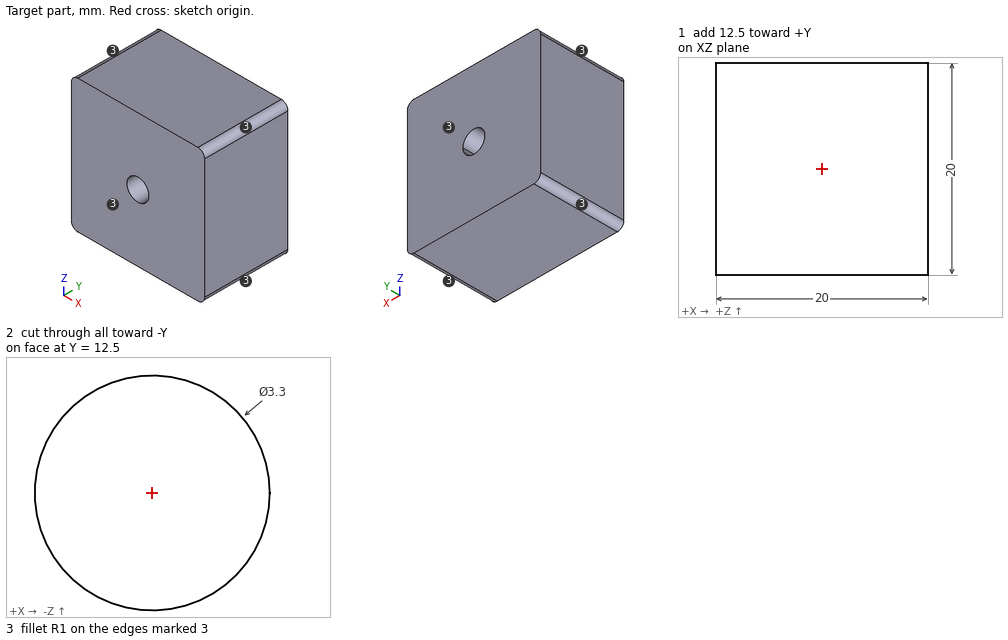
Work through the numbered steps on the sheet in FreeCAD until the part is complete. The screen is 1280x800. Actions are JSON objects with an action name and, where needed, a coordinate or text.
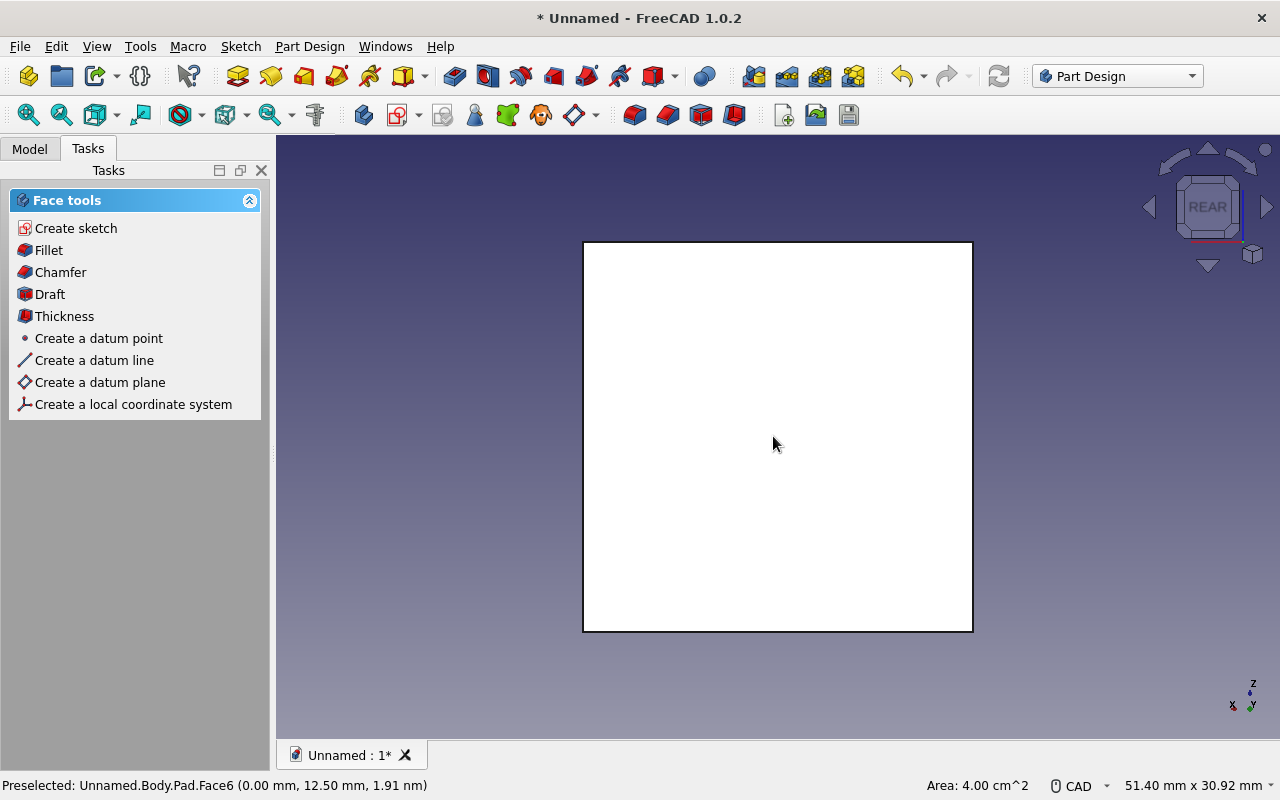
{"action": "left_click", "coordinate": [396, 116]}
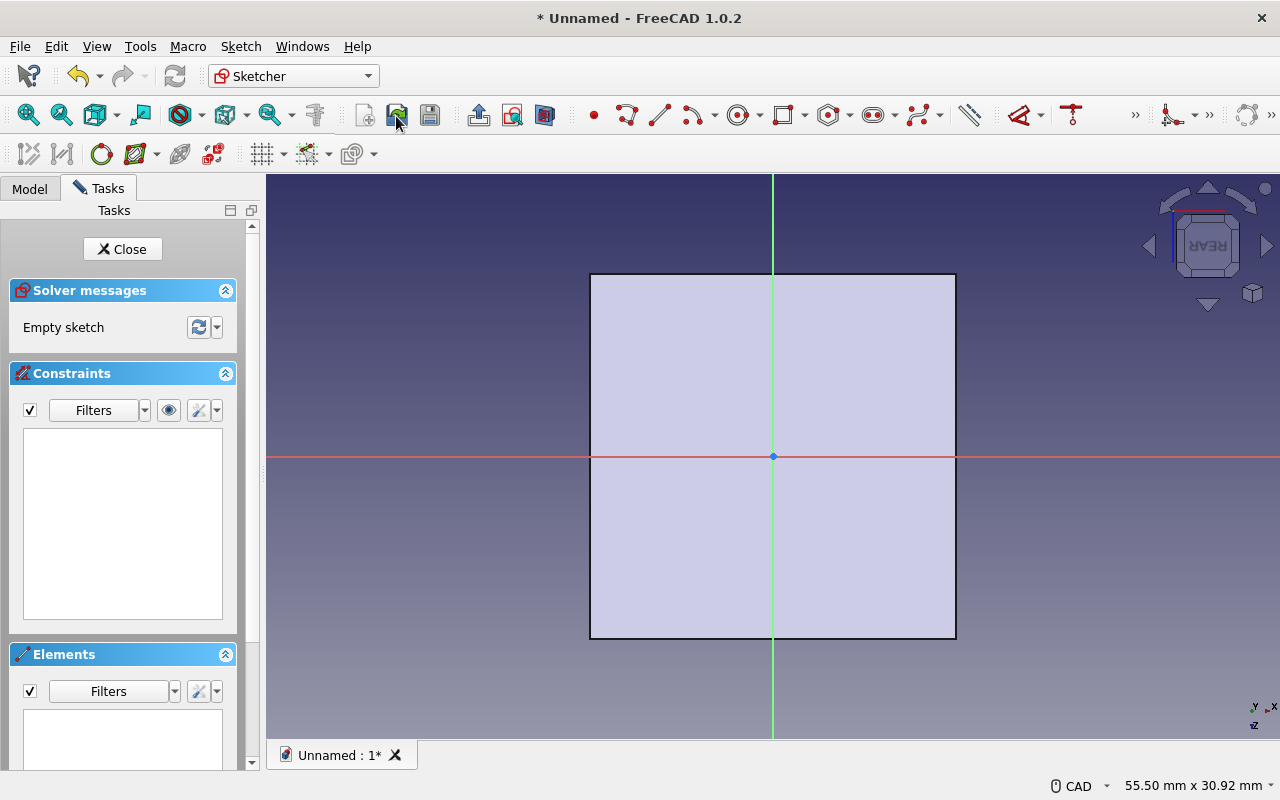
{"action": "scroll", "coordinate": [787, 456], "scroll_direction": "up", "scroll_amount": 9}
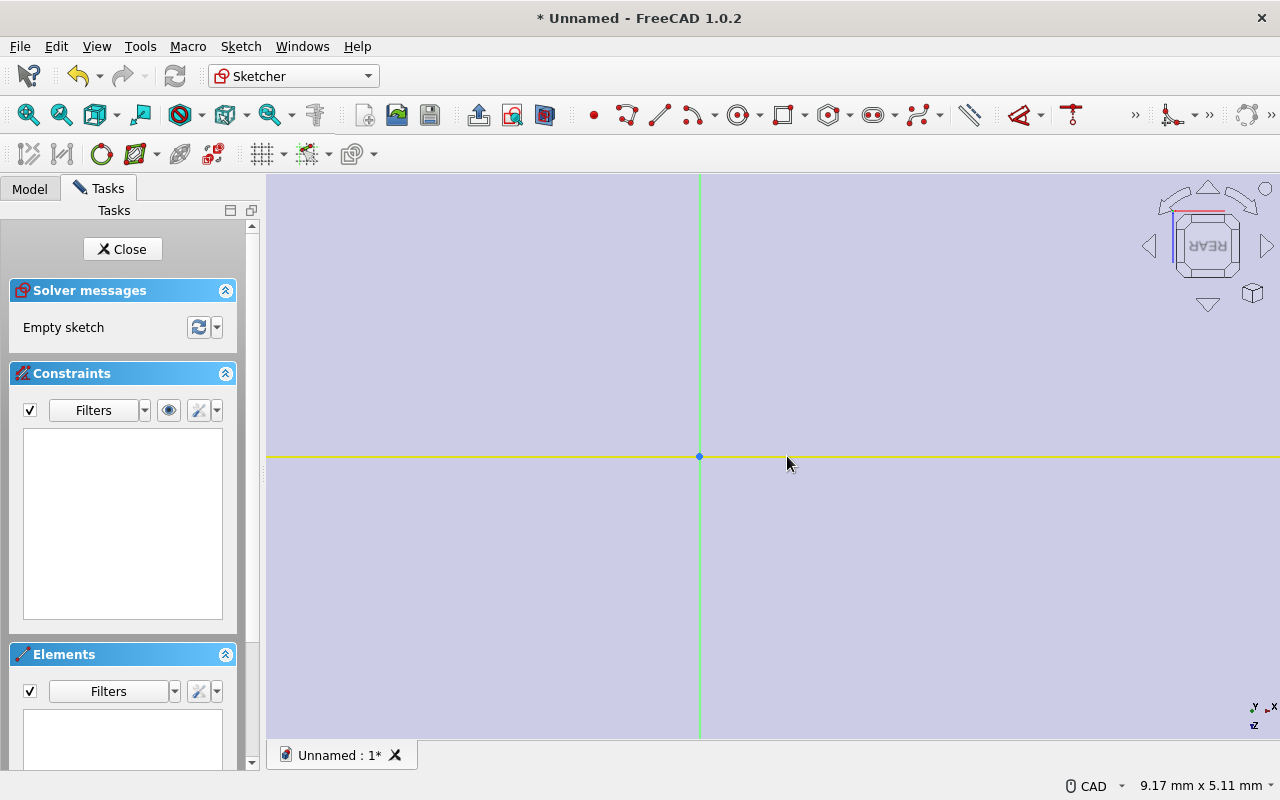
{"action": "left_click", "coordinate": [738, 116]}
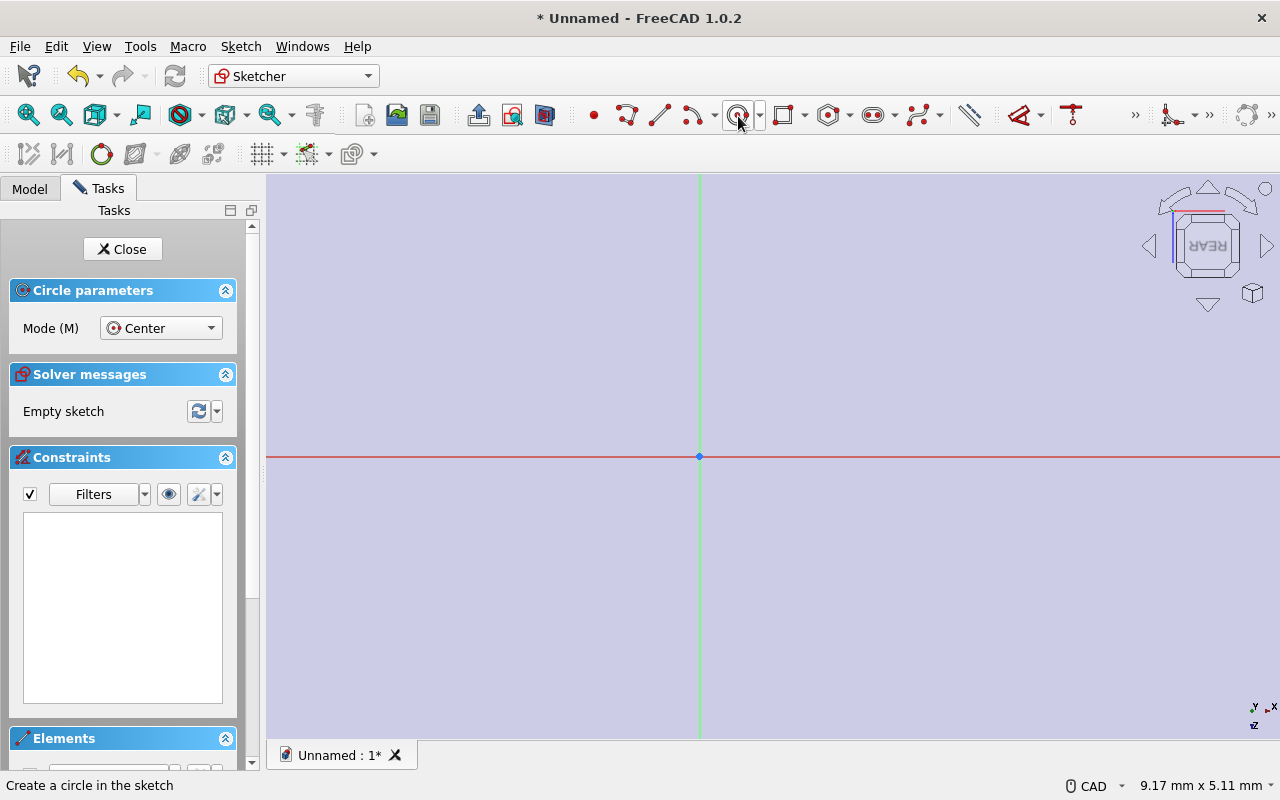
{"action": "left_click", "coordinate": [700, 456]}
{"action": "left_click", "coordinate": [829, 328]}
{"action": "key", "text": "Escape"}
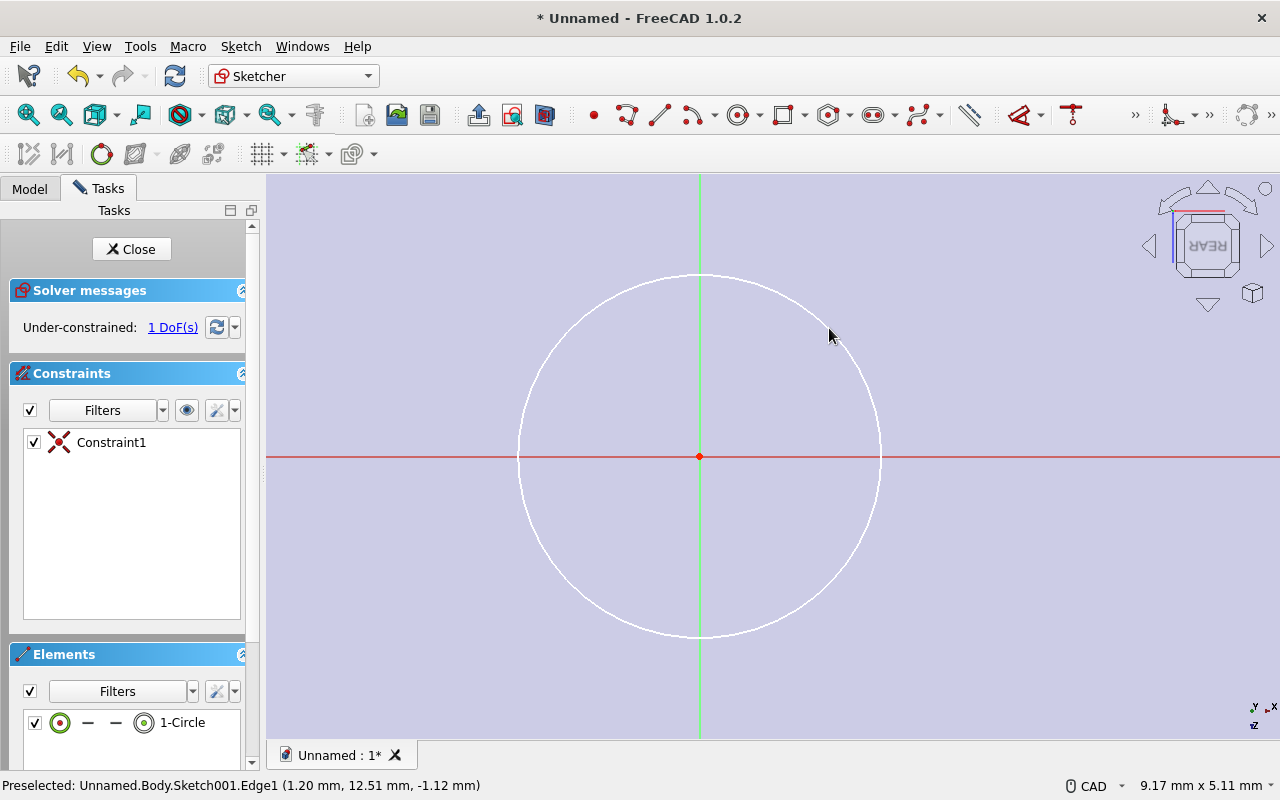
{"action": "left_click", "coordinate": [1018, 116]}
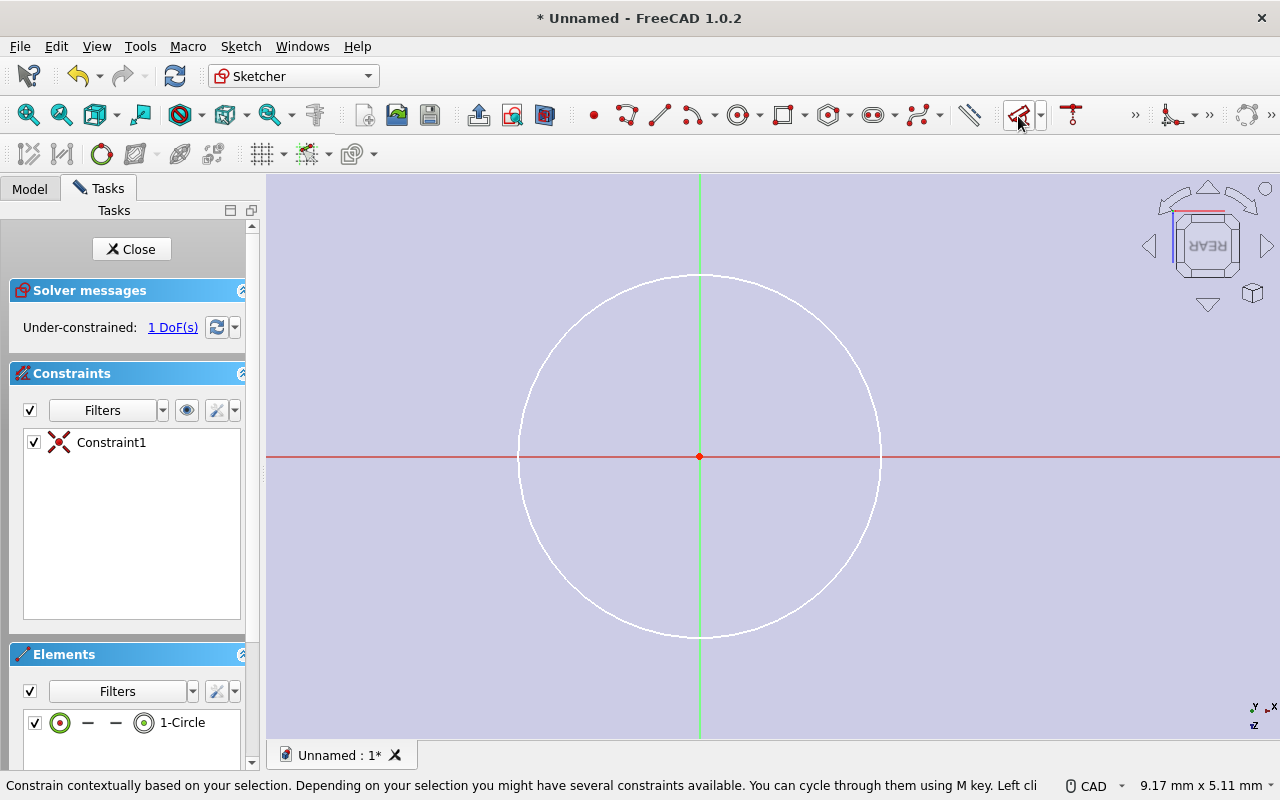
{"action": "left_click", "coordinate": [828, 328]}
{"action": "left_click", "coordinate": [851, 305]}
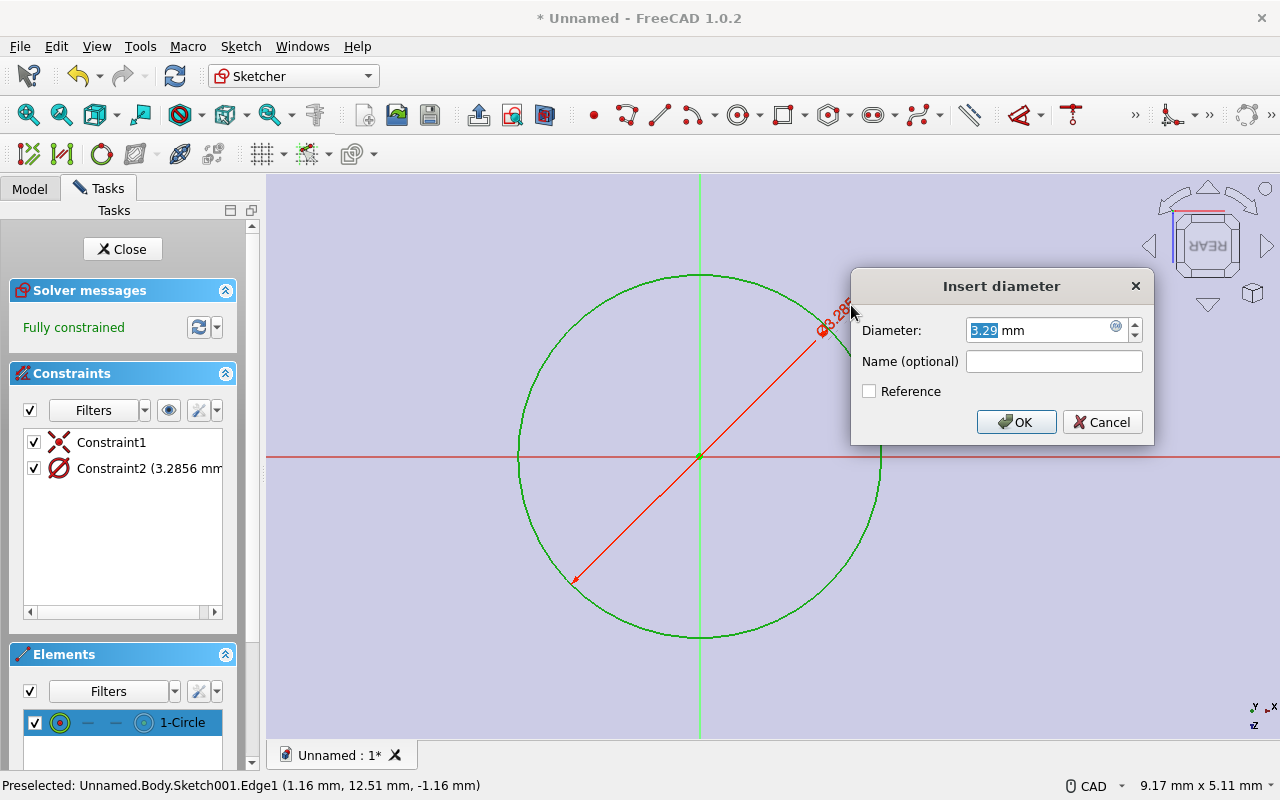
{"action": "type", "text": "3.3"}
{"action": "key", "text": "Return"}
{"action": "key", "text": "Escape"}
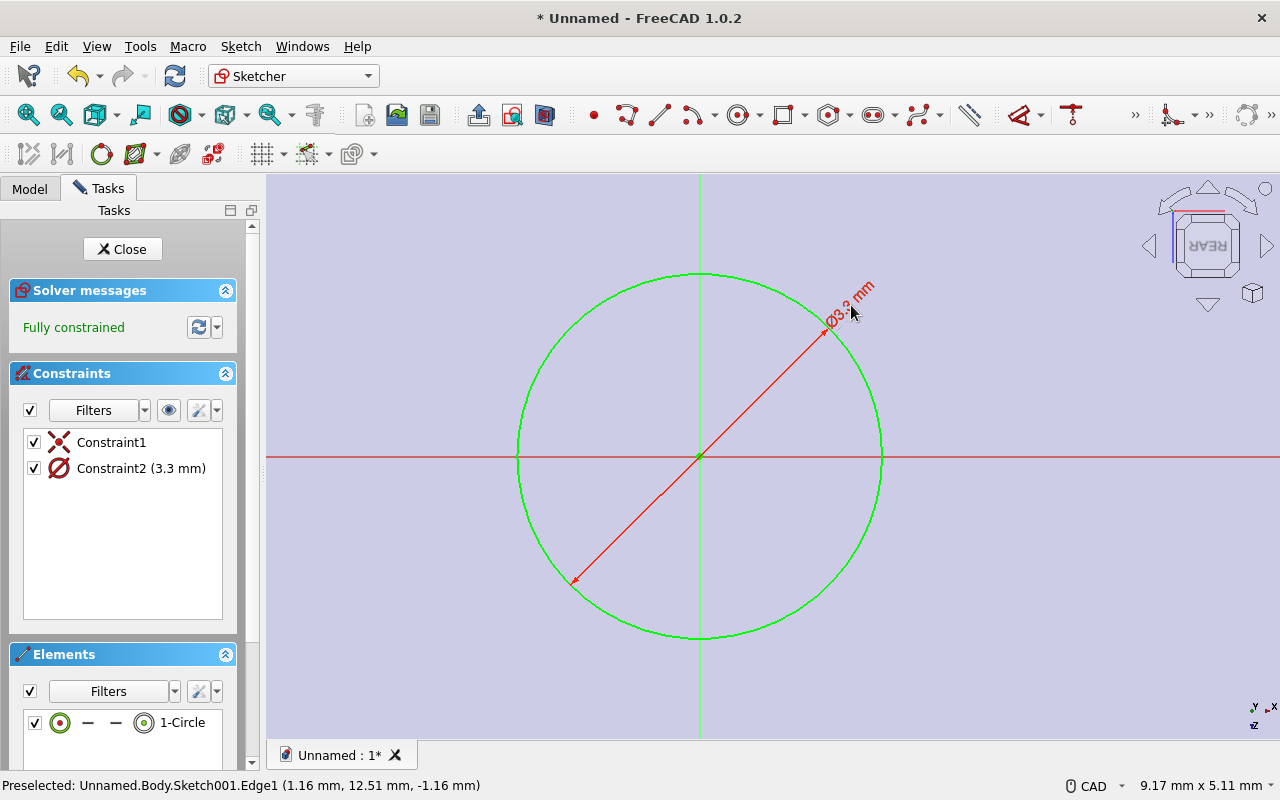
{"action": "left_click", "coordinate": [123, 249]}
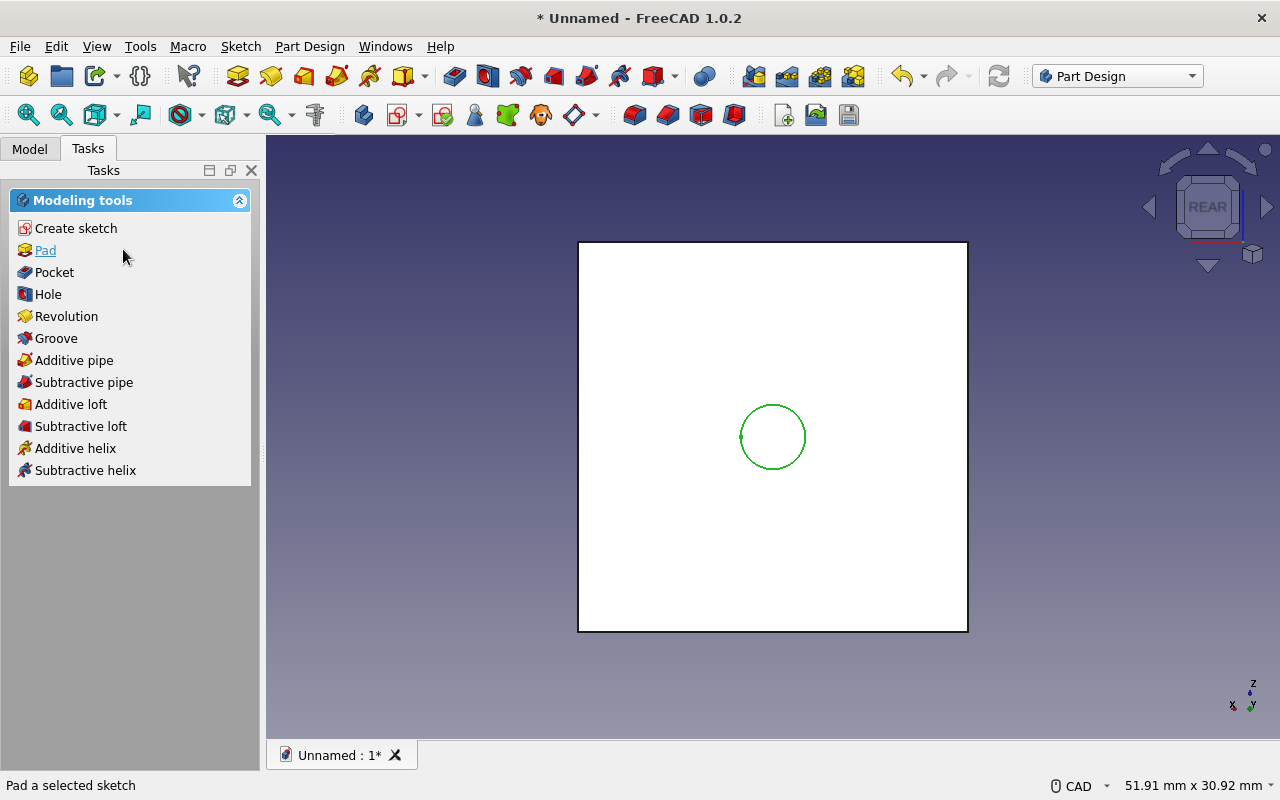
{"action": "left_click", "coordinate": [455, 76]}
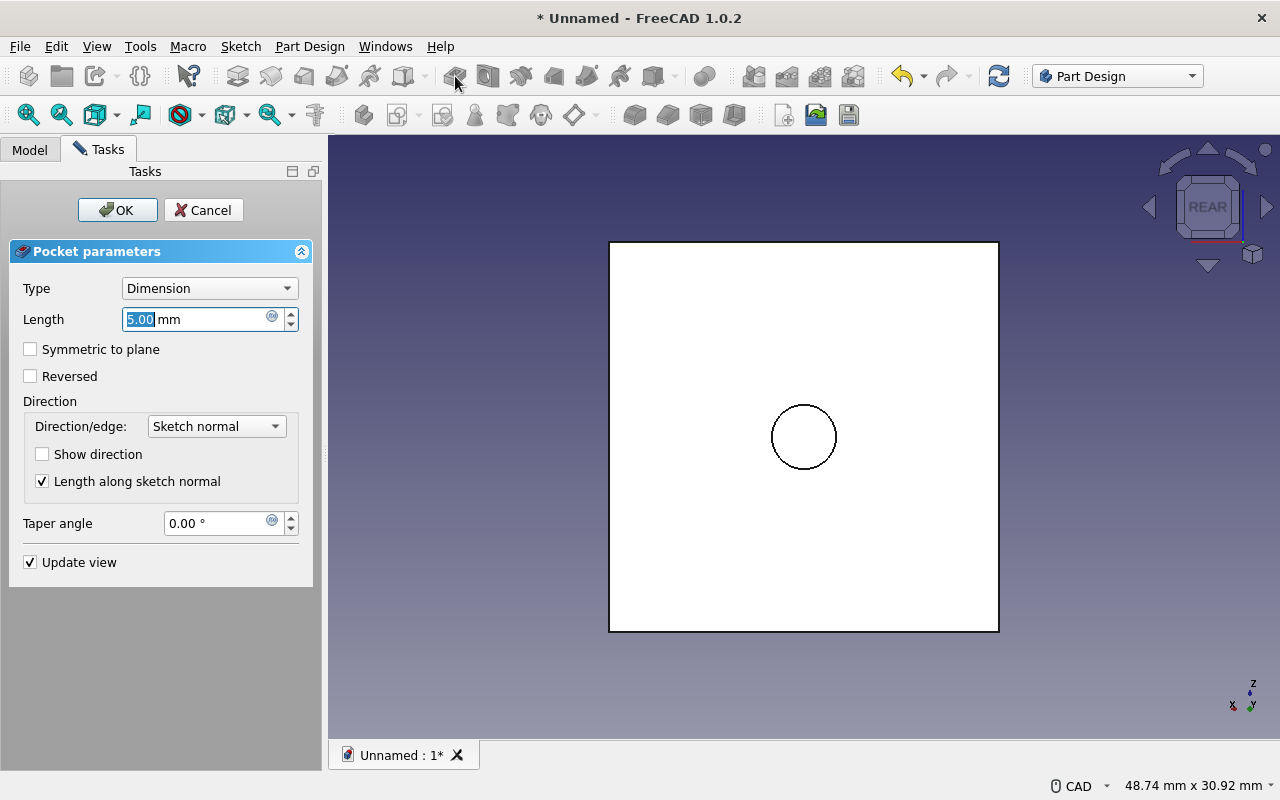
{"action": "left_click", "coordinate": [210, 288]}